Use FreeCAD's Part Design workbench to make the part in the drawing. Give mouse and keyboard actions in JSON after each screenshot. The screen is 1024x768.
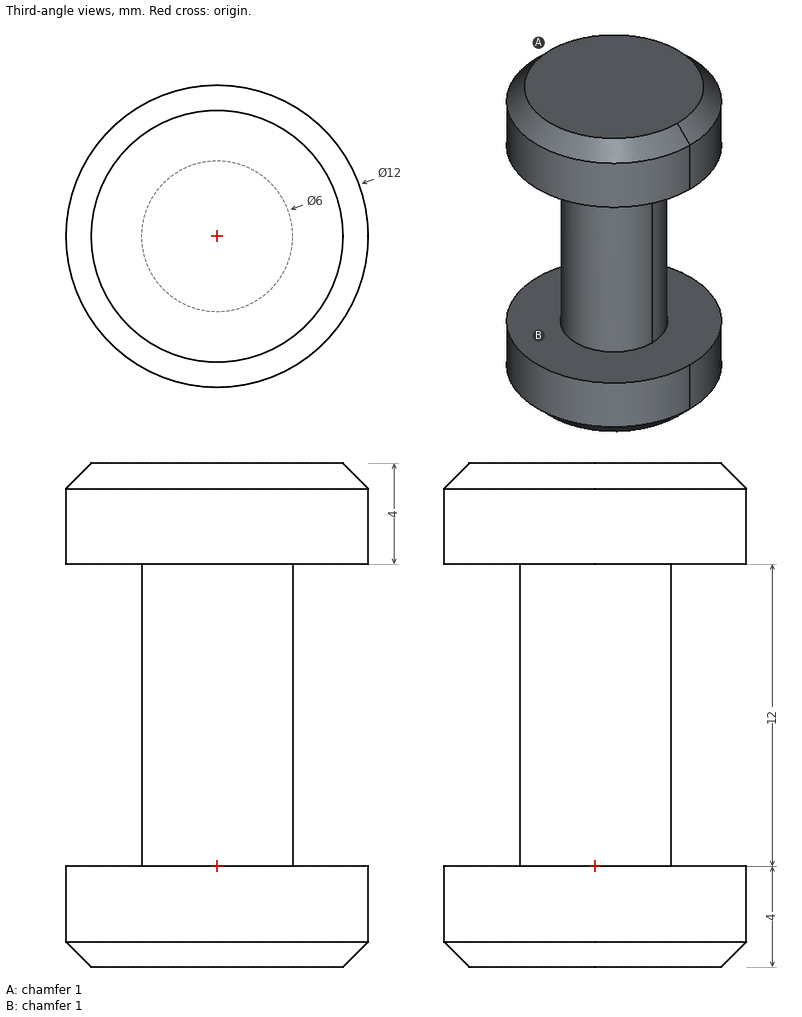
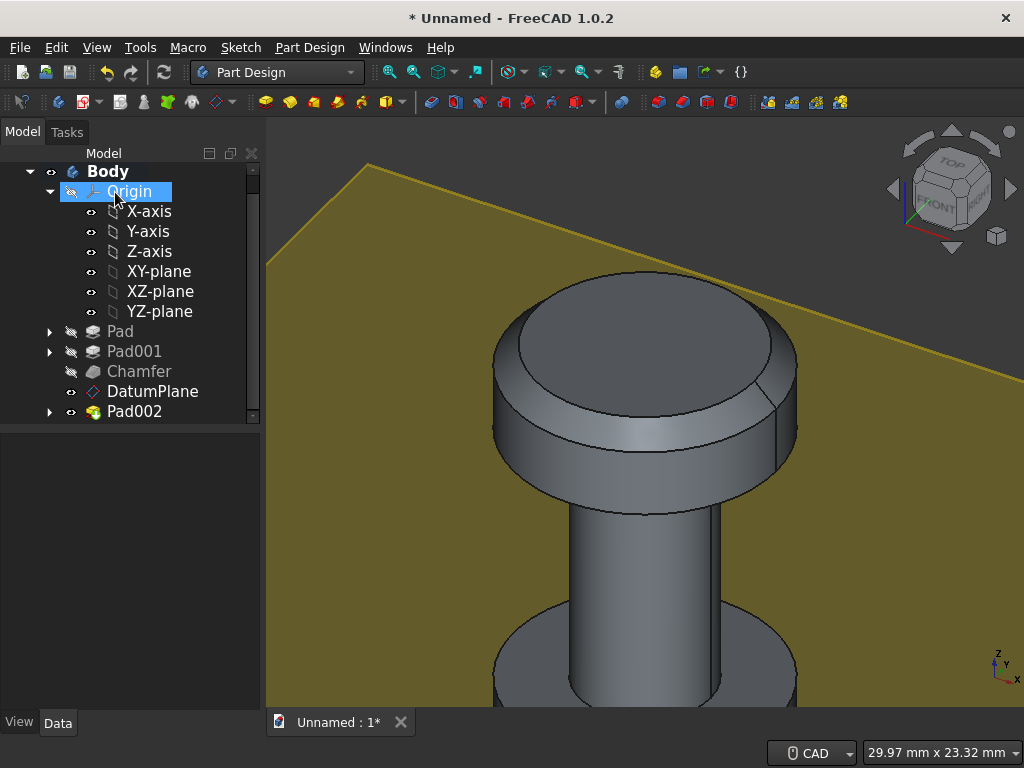
{"action": "left_click", "coordinate": [116, 392]}
{"action": "key", "text": "space"}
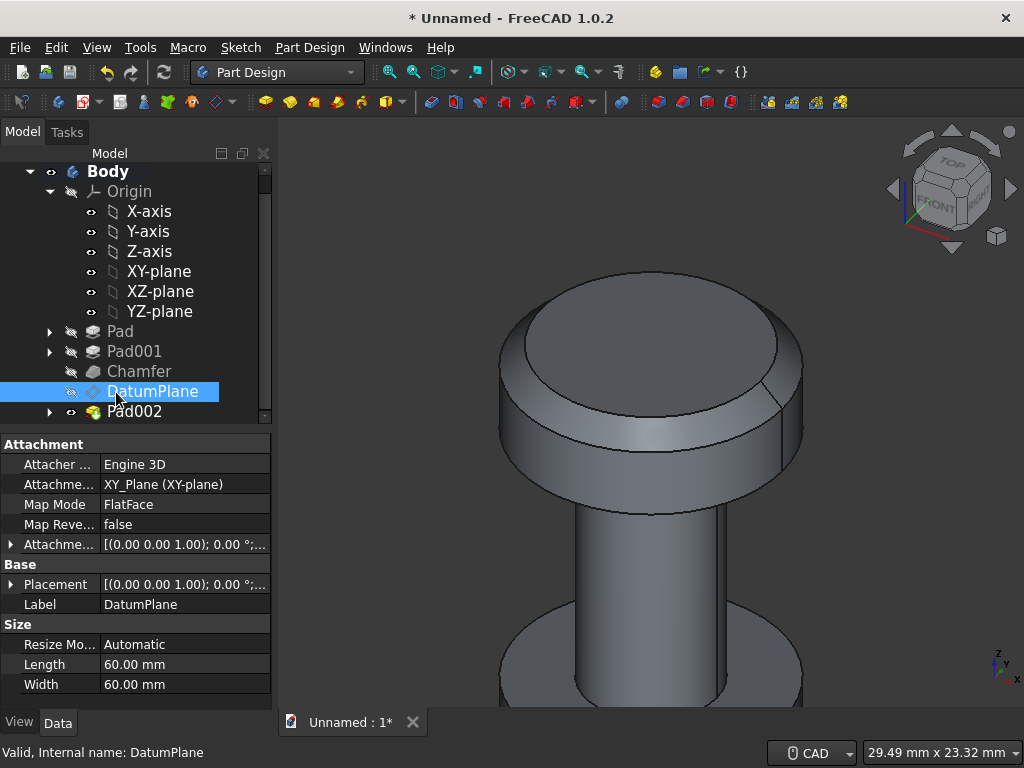
{"action": "left_click", "coordinate": [390, 72]}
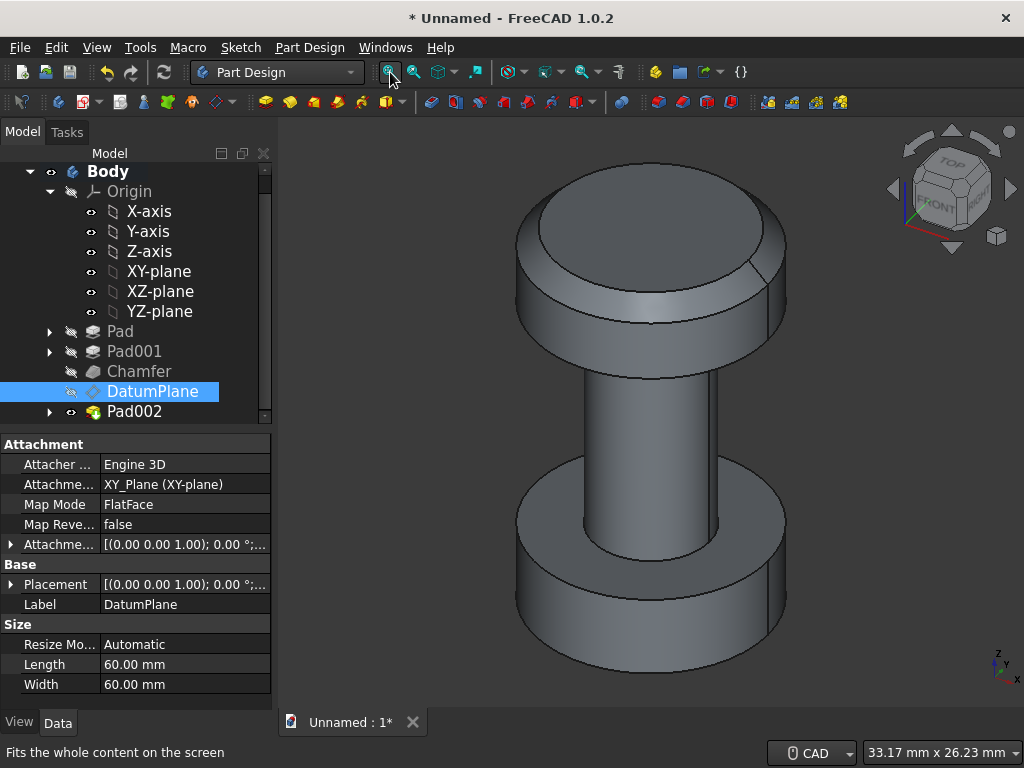
{"action": "key", "text": "0"}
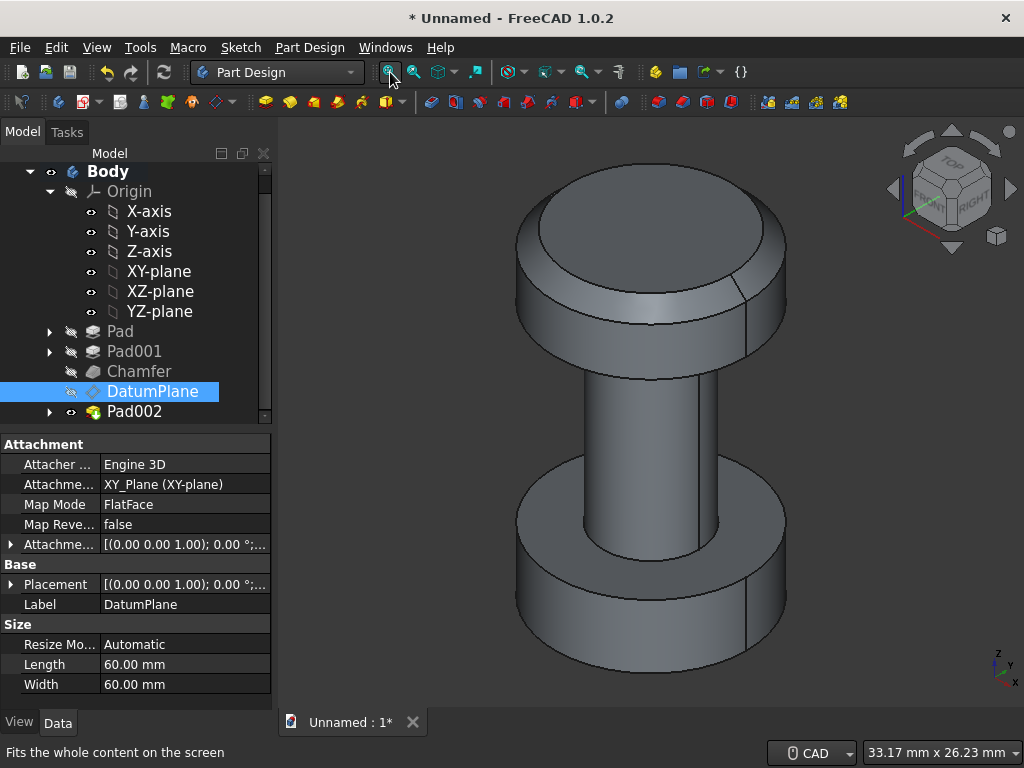
{"action": "key", "text": "2"}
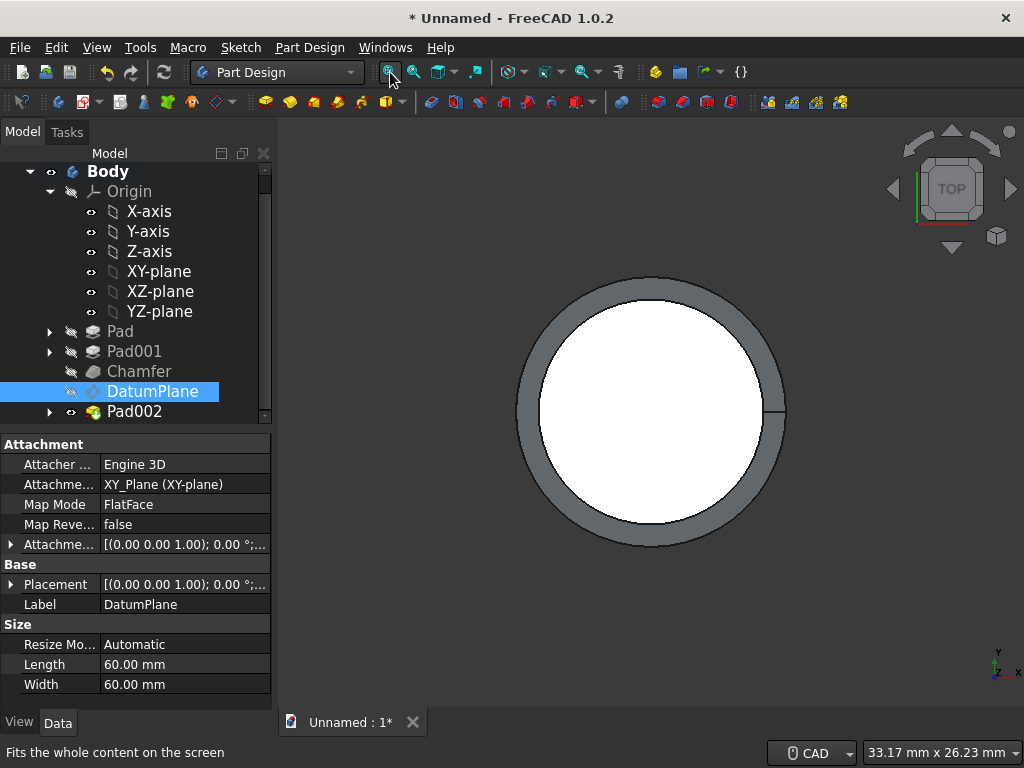
{"action": "key", "text": "1"}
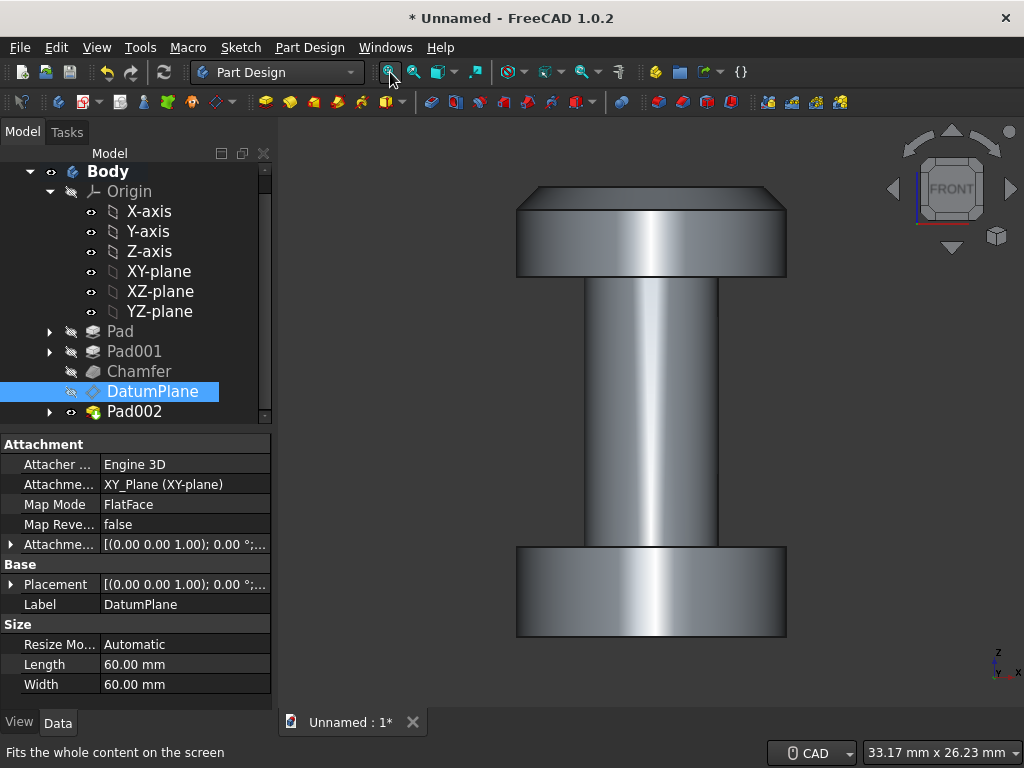
{"action": "left_click", "coordinate": [542, 636]}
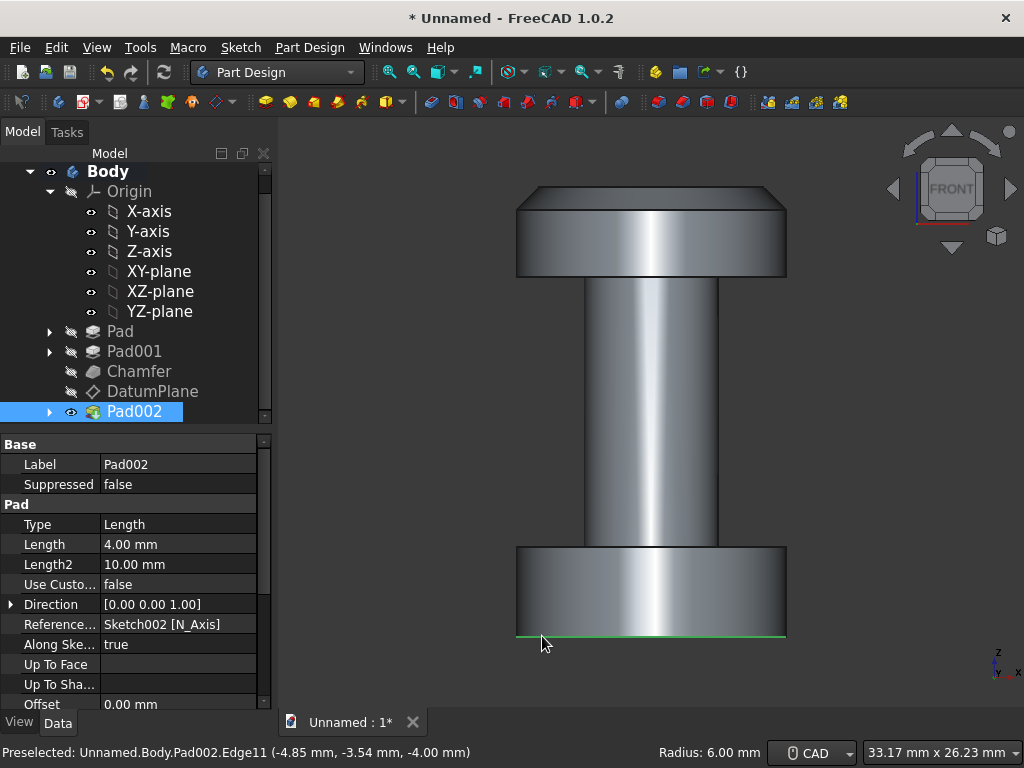
{"action": "left_click", "coordinate": [684, 102]}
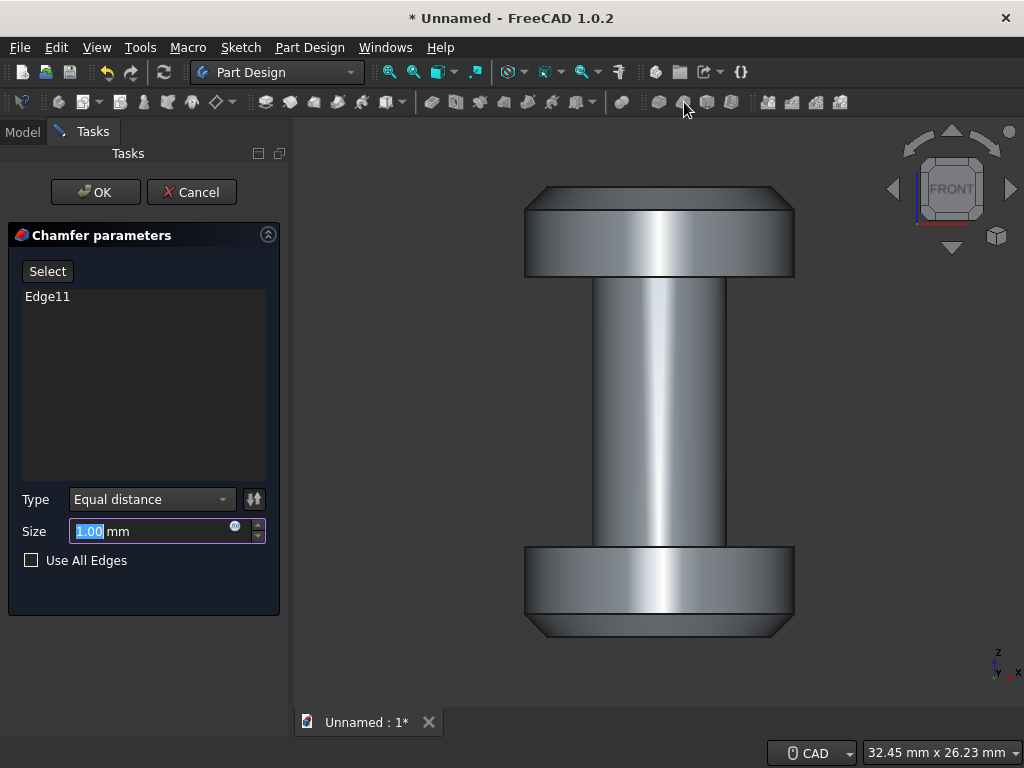
{"action": "type", "text": "1"}
{"action": "key", "text": "Tab"}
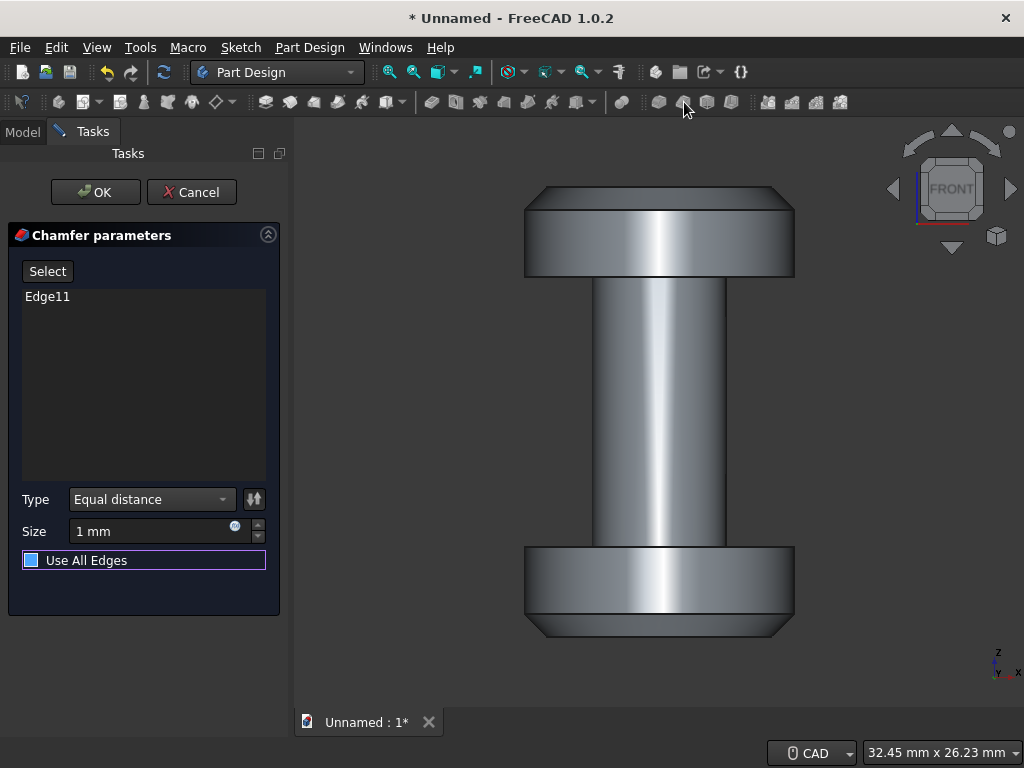
{"action": "left_click", "coordinate": [96, 192]}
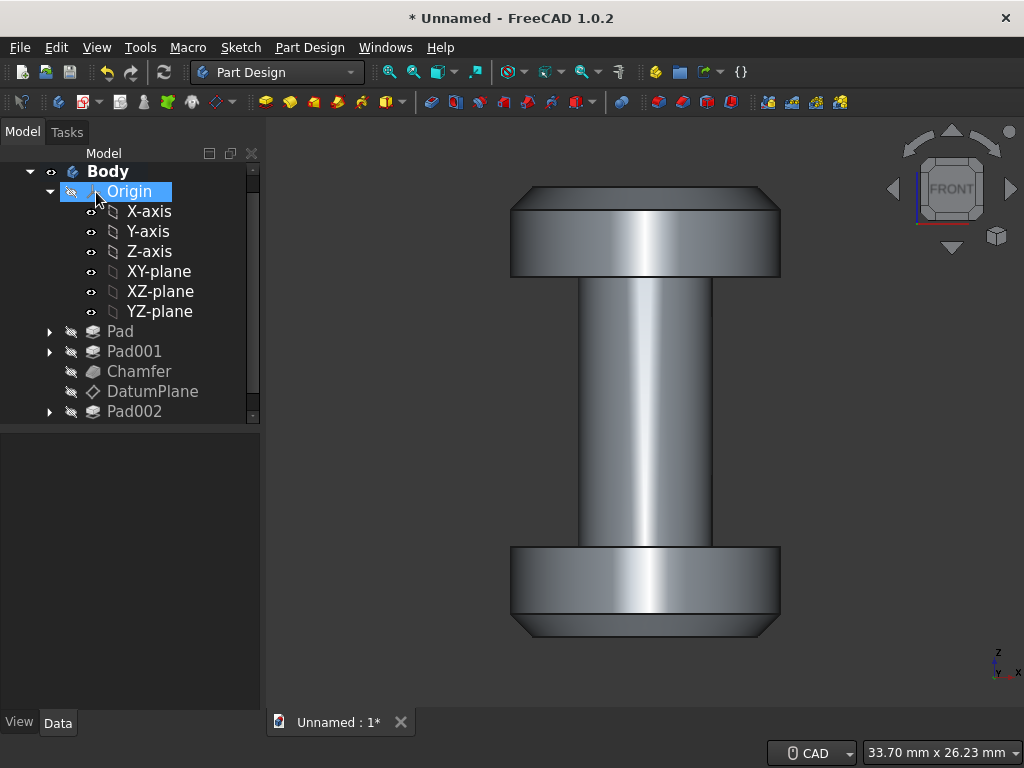
{"action": "key", "text": "0"}